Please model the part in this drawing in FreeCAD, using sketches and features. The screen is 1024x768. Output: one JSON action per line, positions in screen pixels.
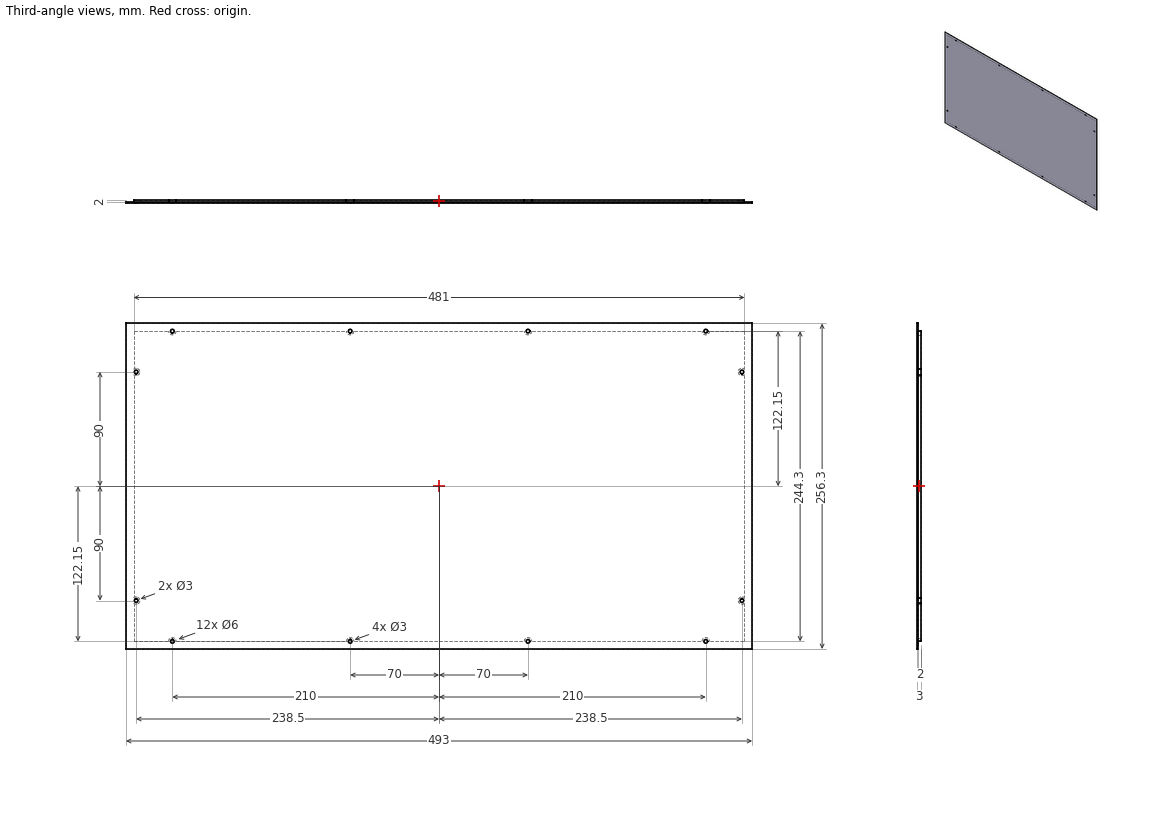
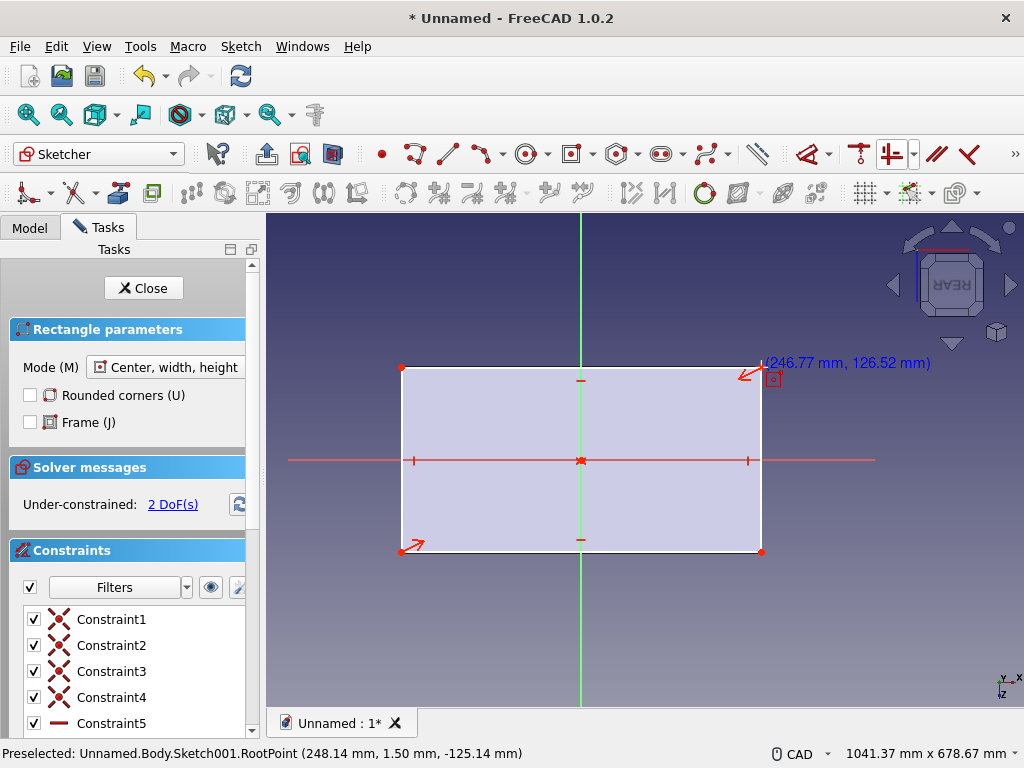
{"action": "left_click", "coordinate": [581, 460]}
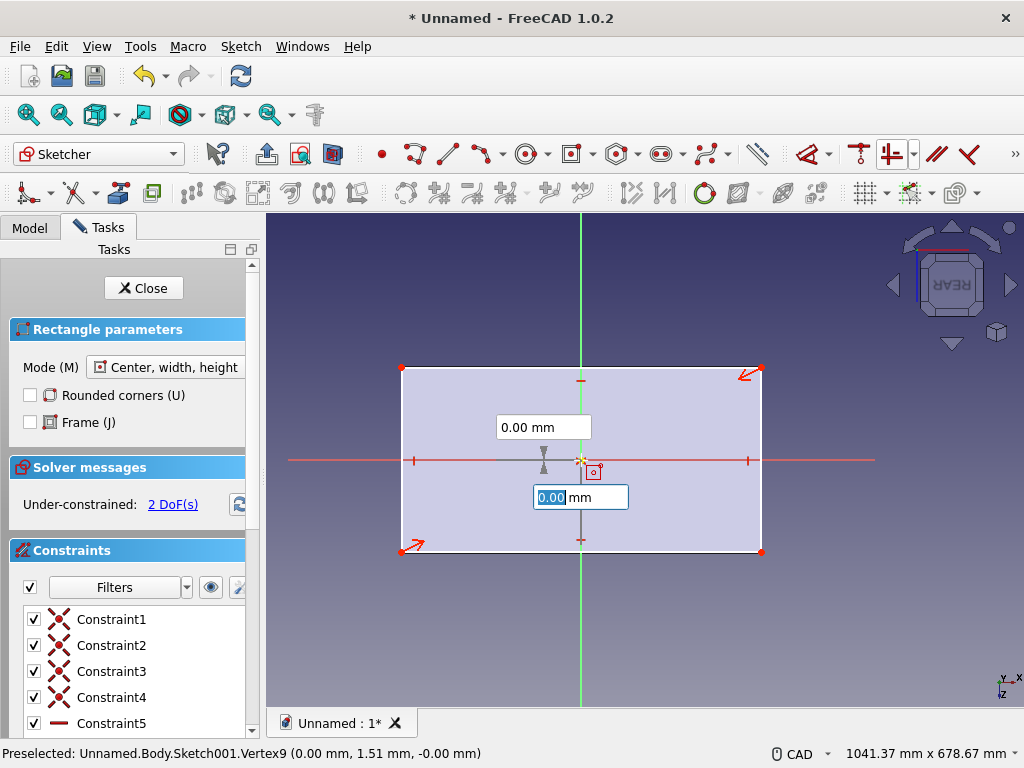
{"action": "scroll", "coordinate": [756, 371], "scroll_direction": "up", "scroll_amount": 7}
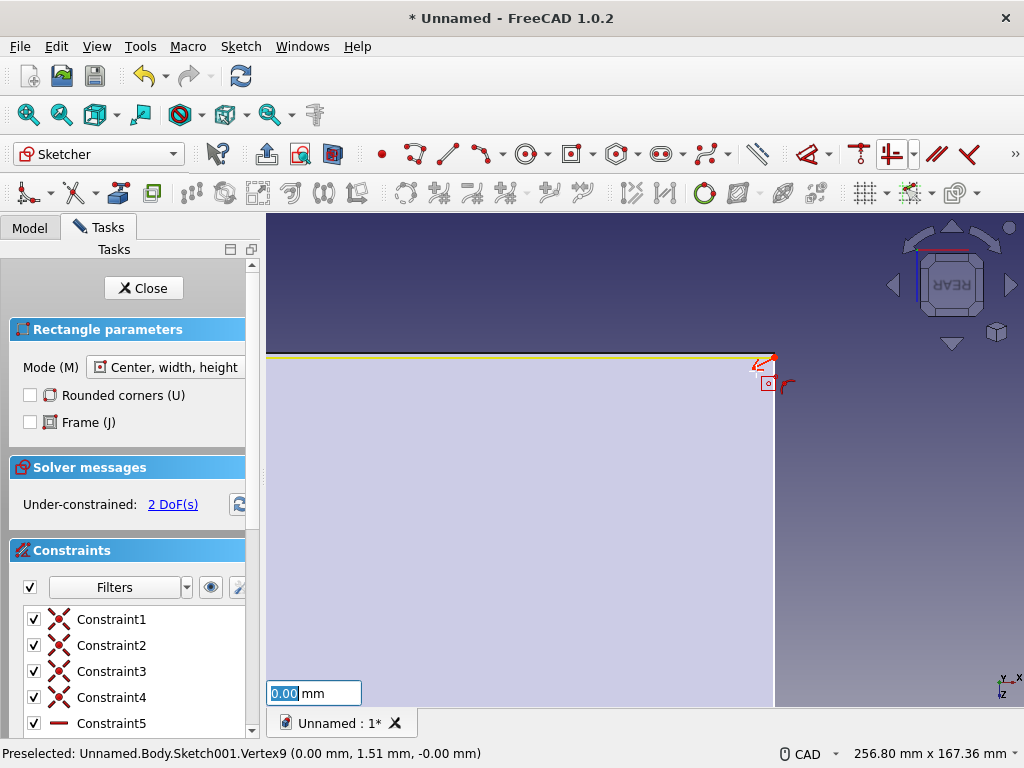
{"action": "left_click", "coordinate": [756, 371]}
{"action": "key", "text": "Escape"}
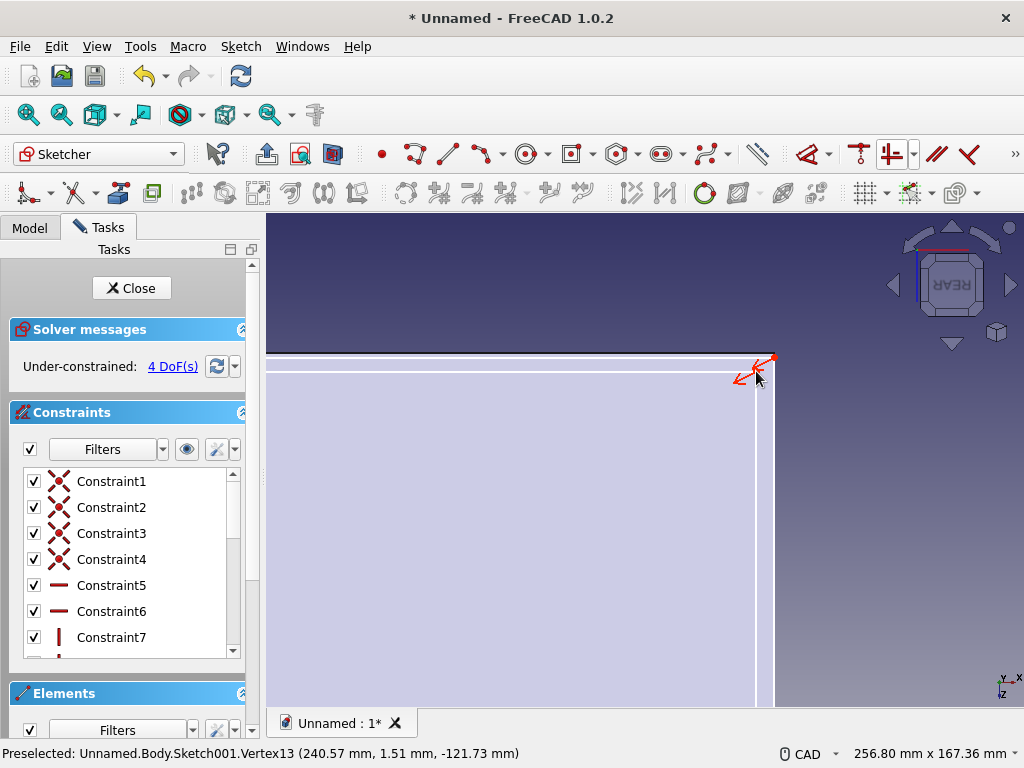
{"action": "left_click", "coordinate": [806, 154]}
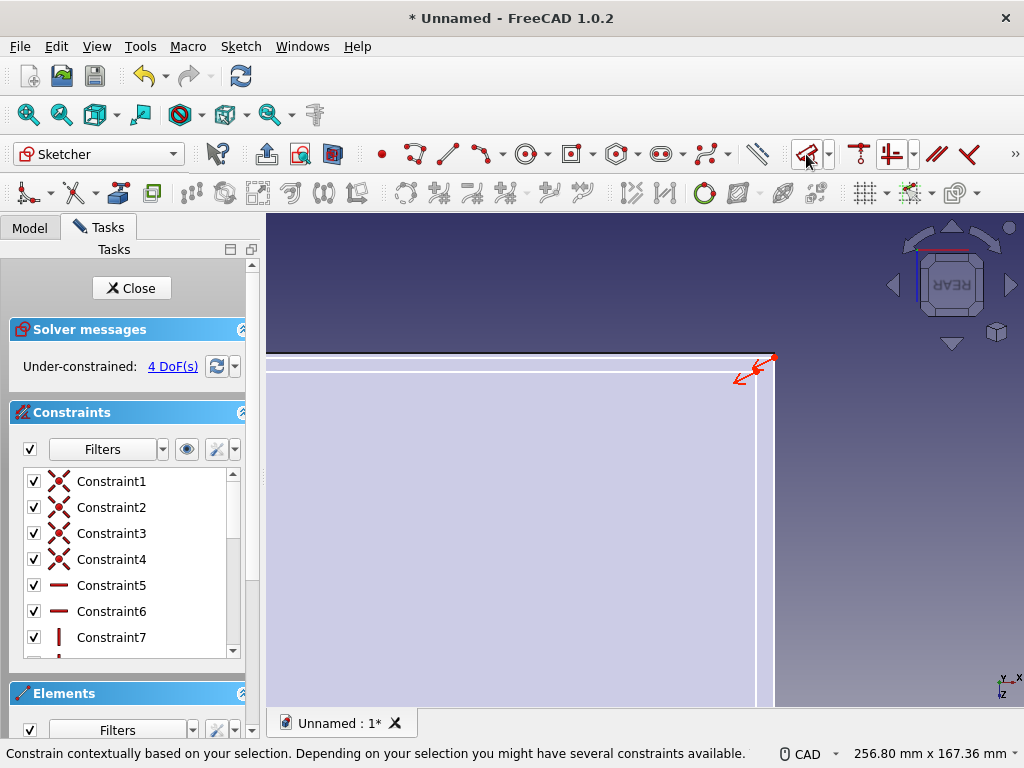
{"action": "scroll", "coordinate": [805, 343], "scroll_direction": "down", "scroll_amount": 6}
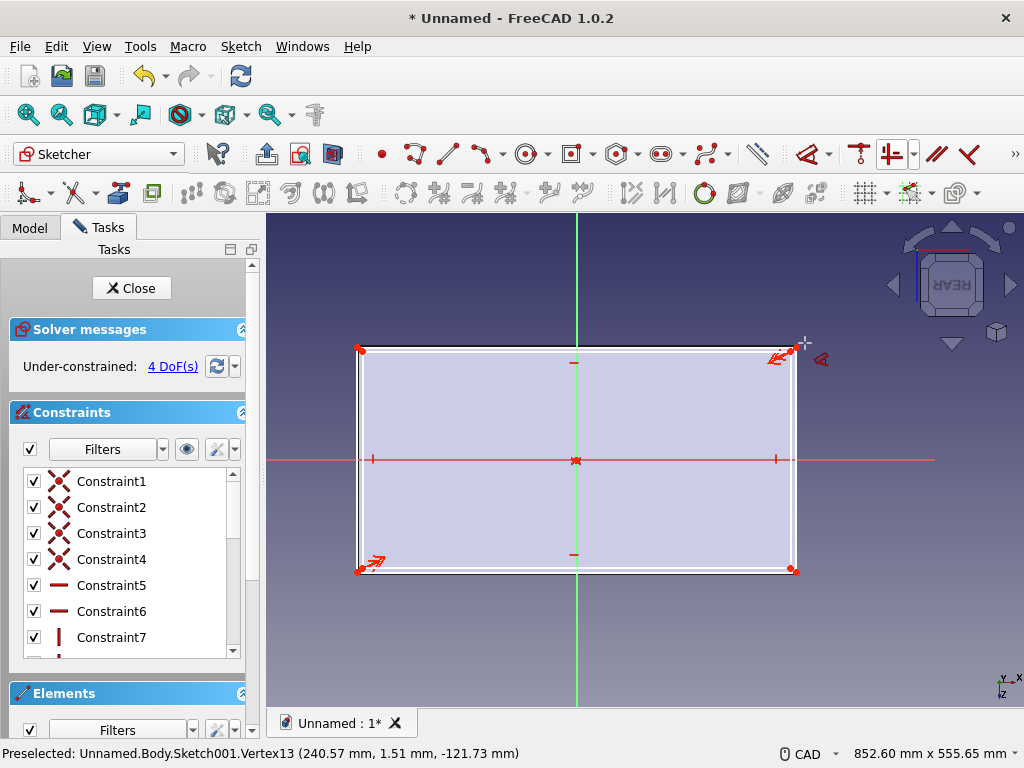
{"action": "scroll", "coordinate": [489, 573], "scroll_direction": "up", "scroll_amount": 6}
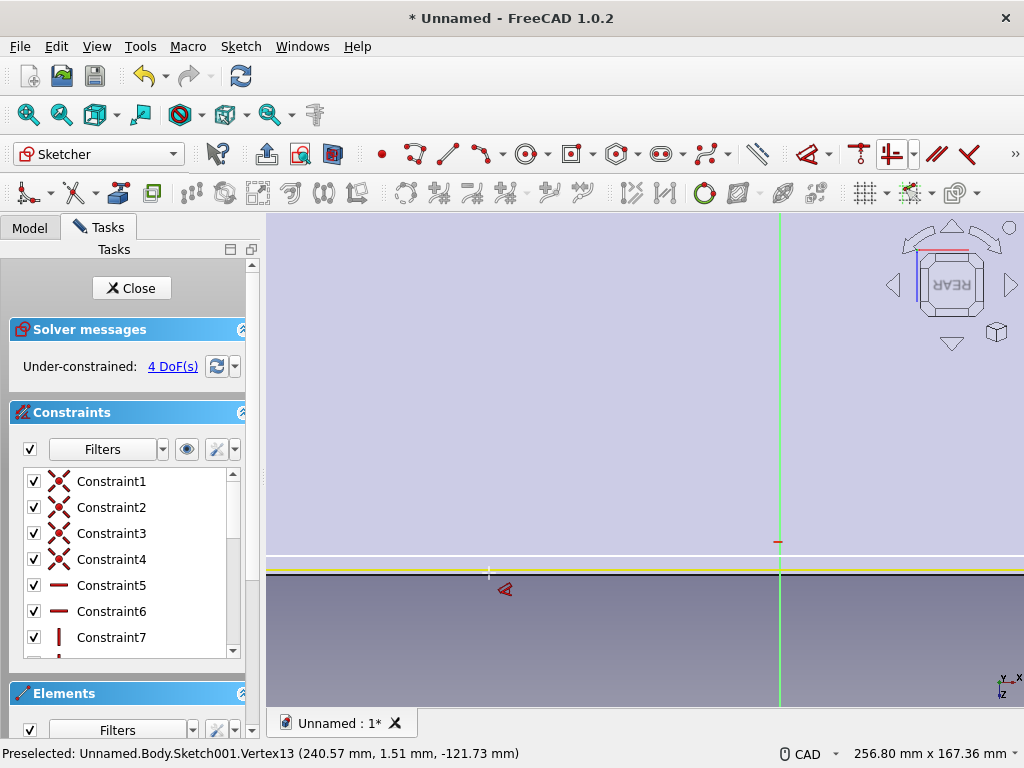
{"action": "left_click", "coordinate": [489, 570]}
{"action": "left_click", "coordinate": [576, 604]}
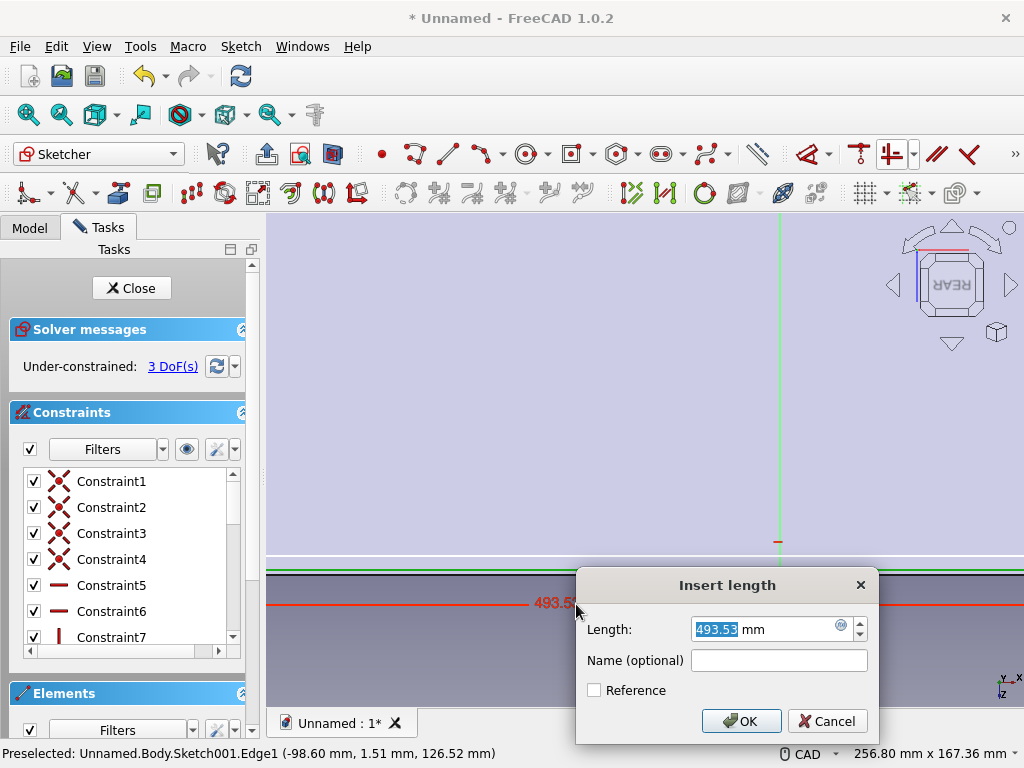
{"action": "type", "text": "493"}
{"action": "key", "text": "Return"}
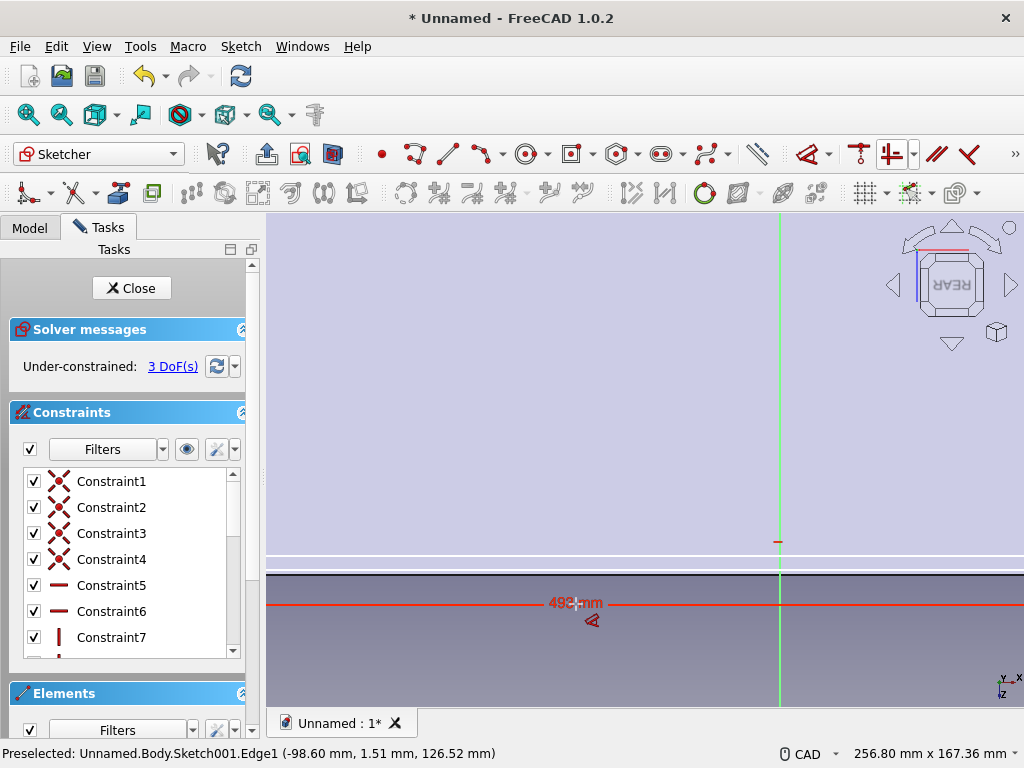
{"action": "left_click", "coordinate": [496, 556]}
{"action": "left_click", "coordinate": [447, 590]}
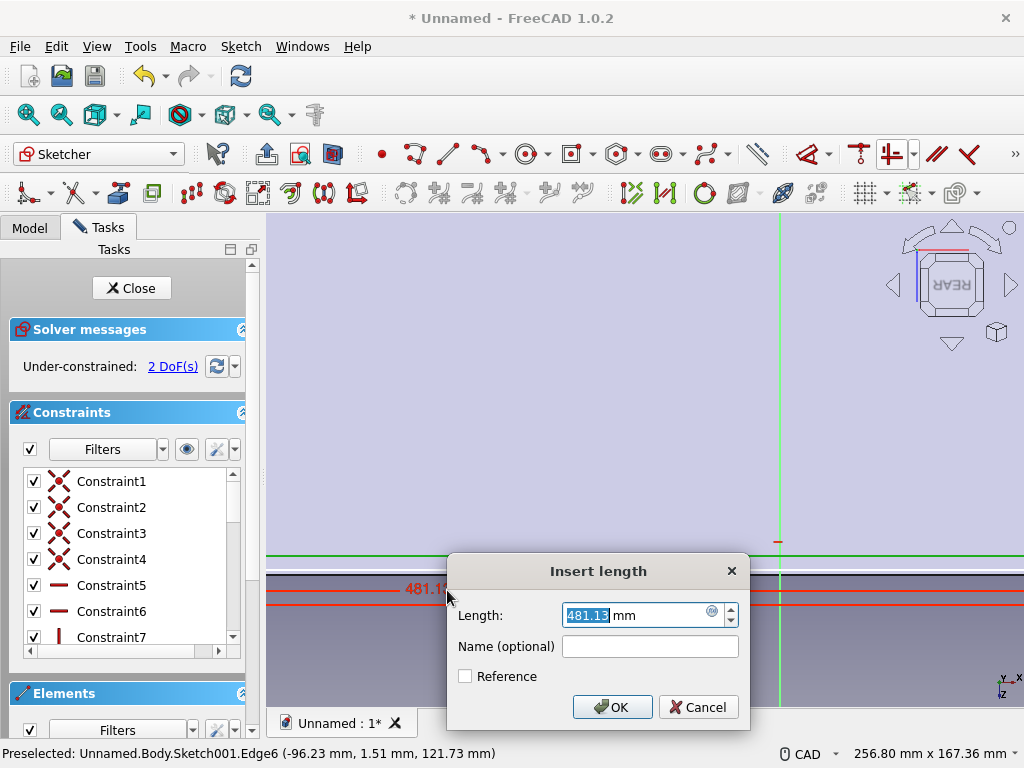
{"action": "type", "text": "481"}
{"action": "key", "text": "Return"}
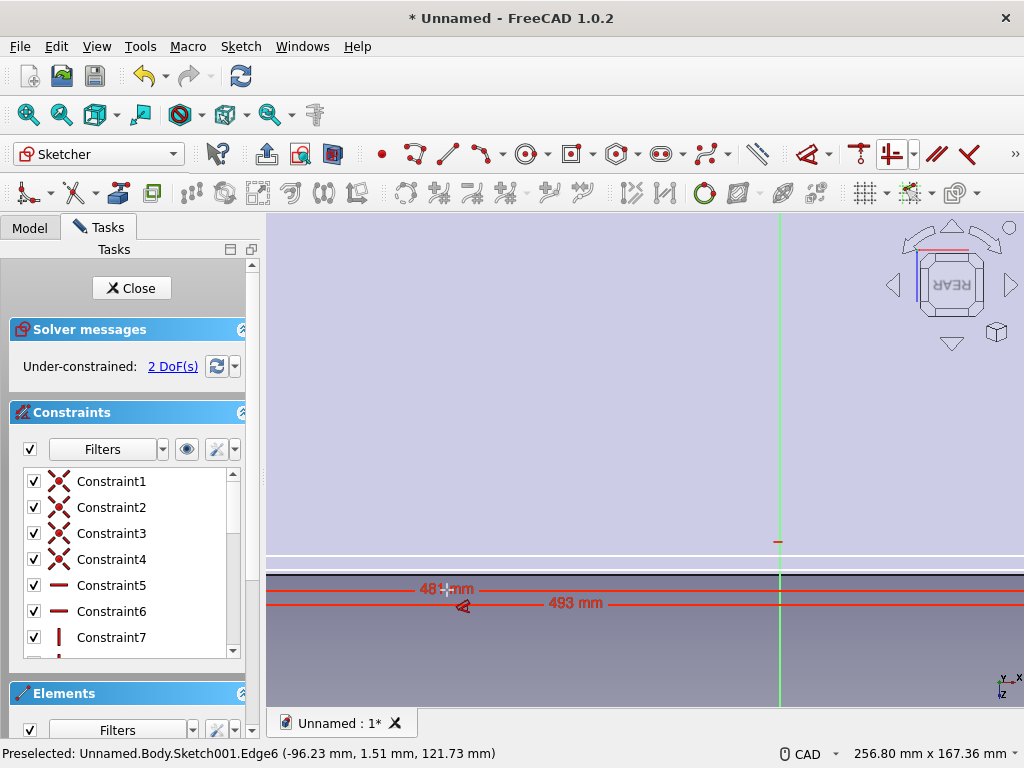
{"action": "scroll", "coordinate": [489, 574], "scroll_direction": "down", "scroll_amount": 6}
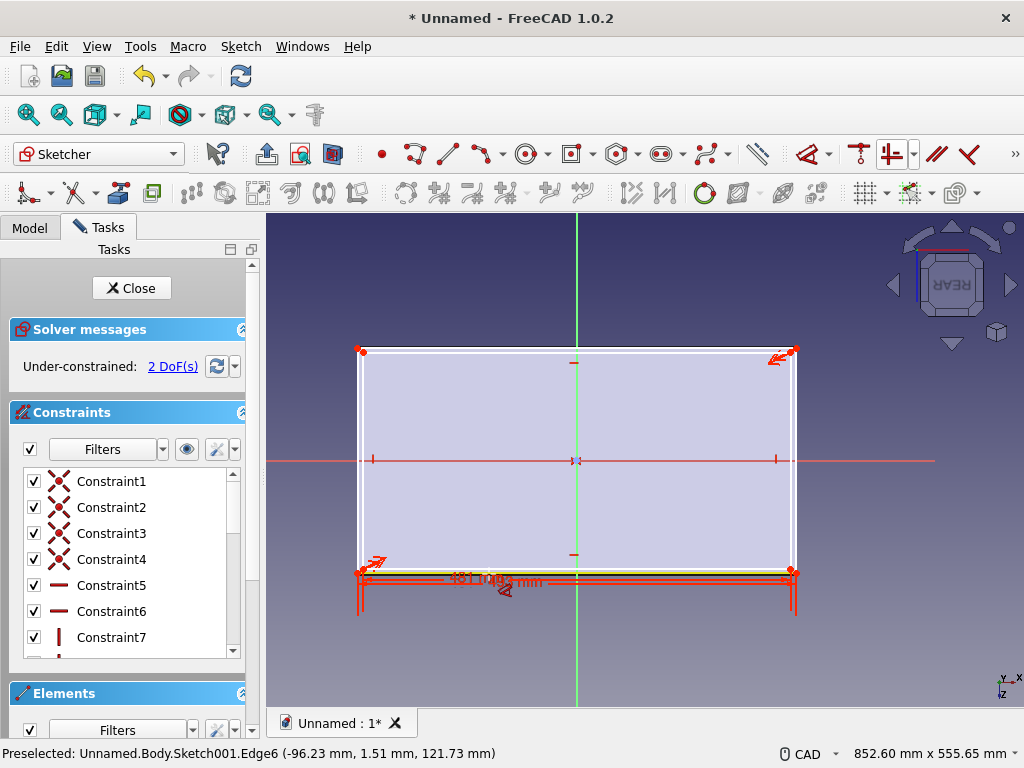
{"action": "scroll", "coordinate": [796, 506], "scroll_direction": "up", "scroll_amount": 5}